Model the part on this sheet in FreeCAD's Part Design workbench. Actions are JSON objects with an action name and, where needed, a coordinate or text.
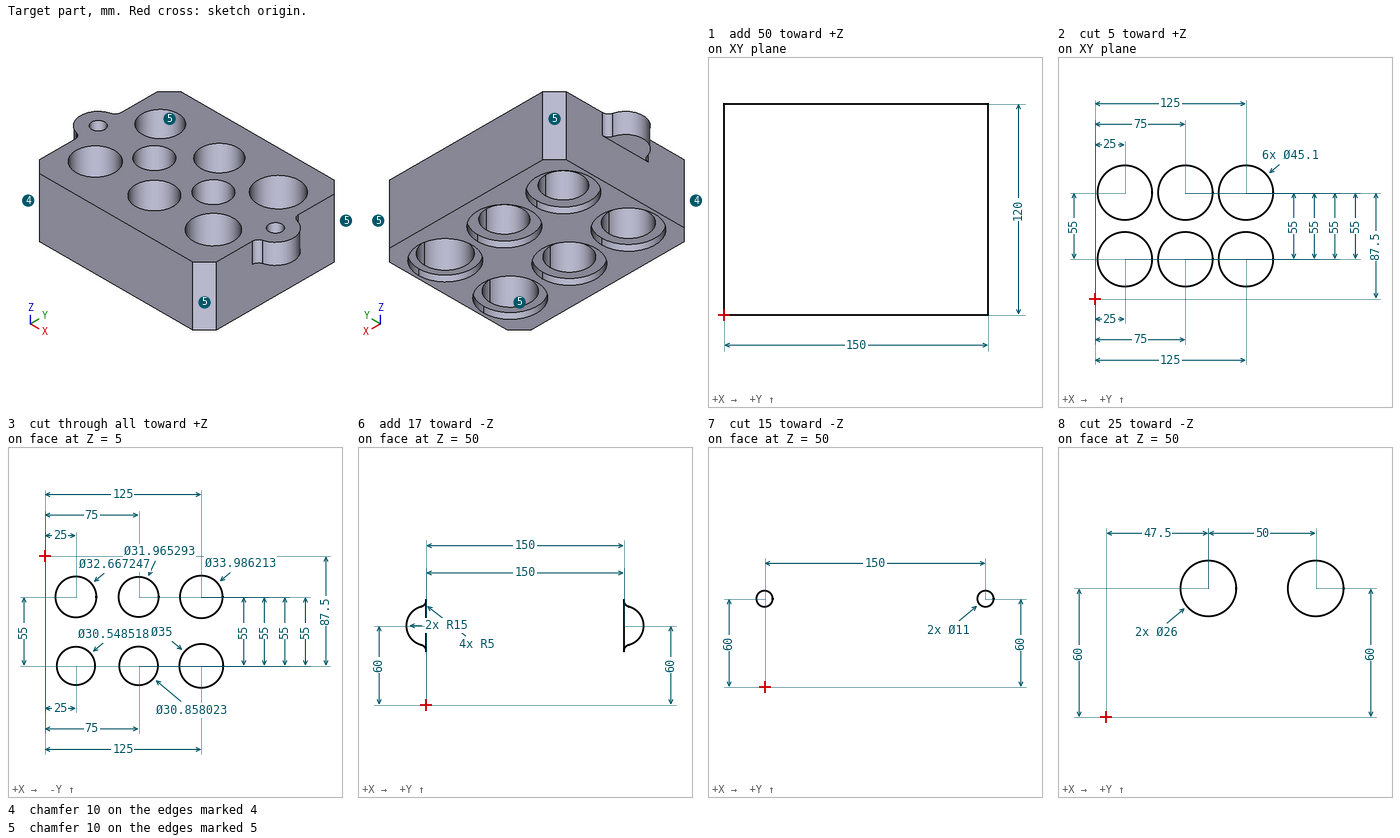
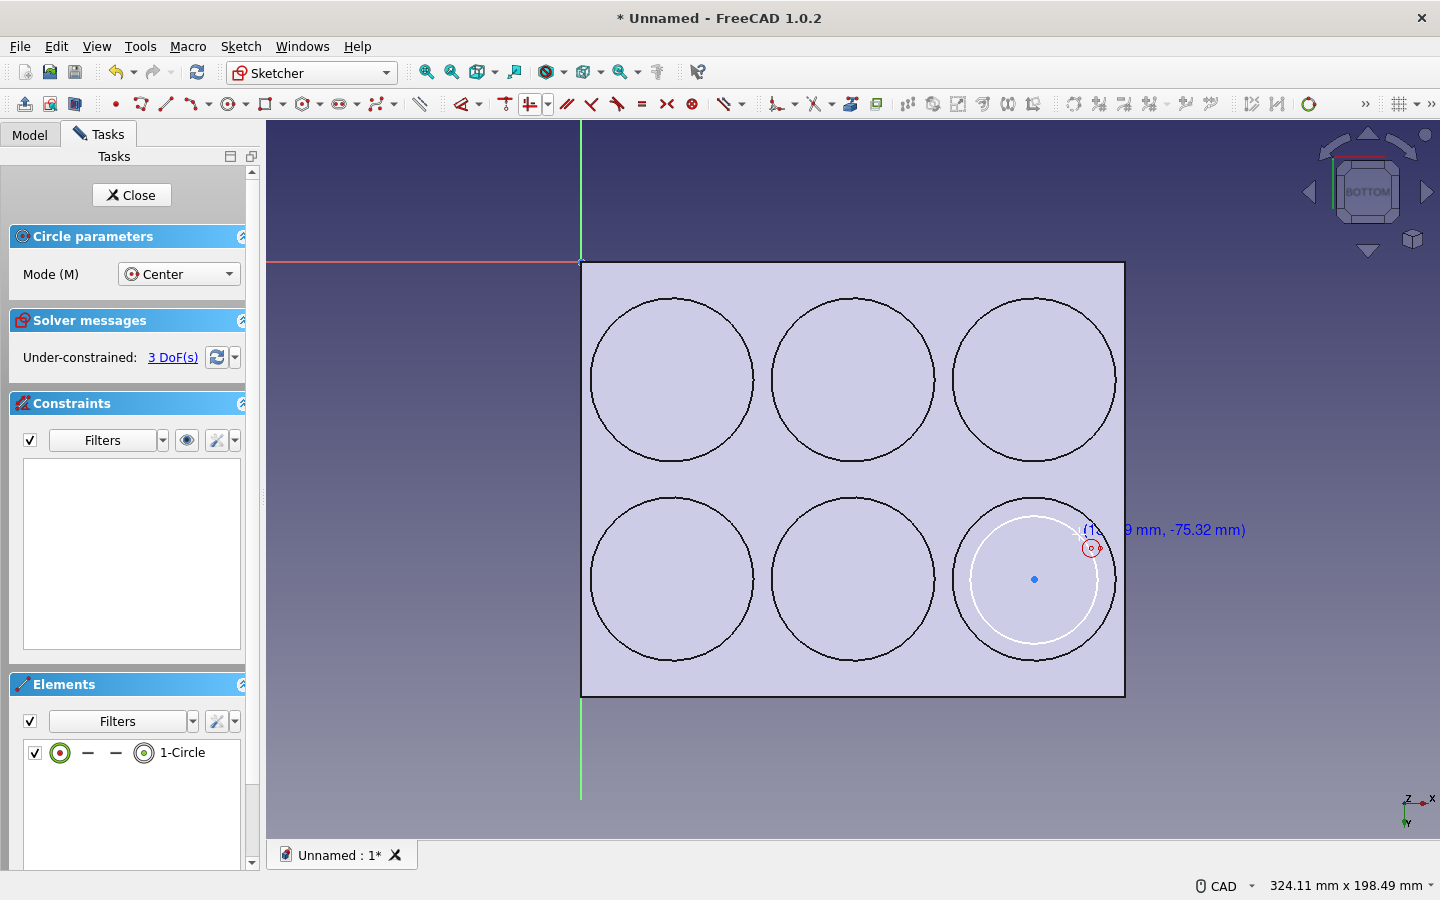
{"action": "left_click", "coordinate": [853, 579]}
{"action": "left_click", "coordinate": [893, 540]}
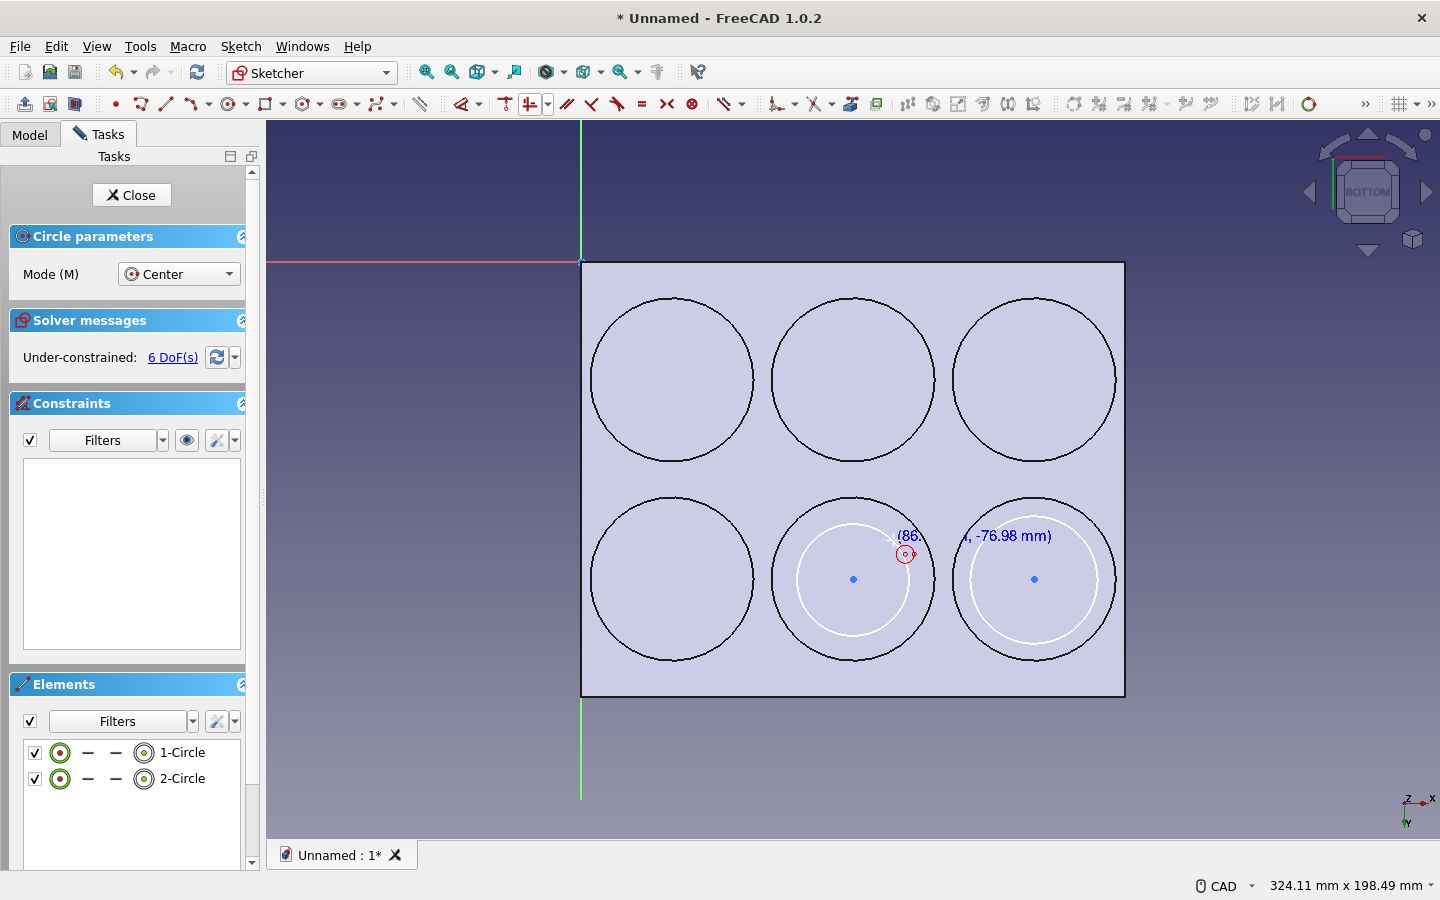
{"action": "left_click", "coordinate": [672, 579]}
{"action": "left_click", "coordinate": [711, 540]}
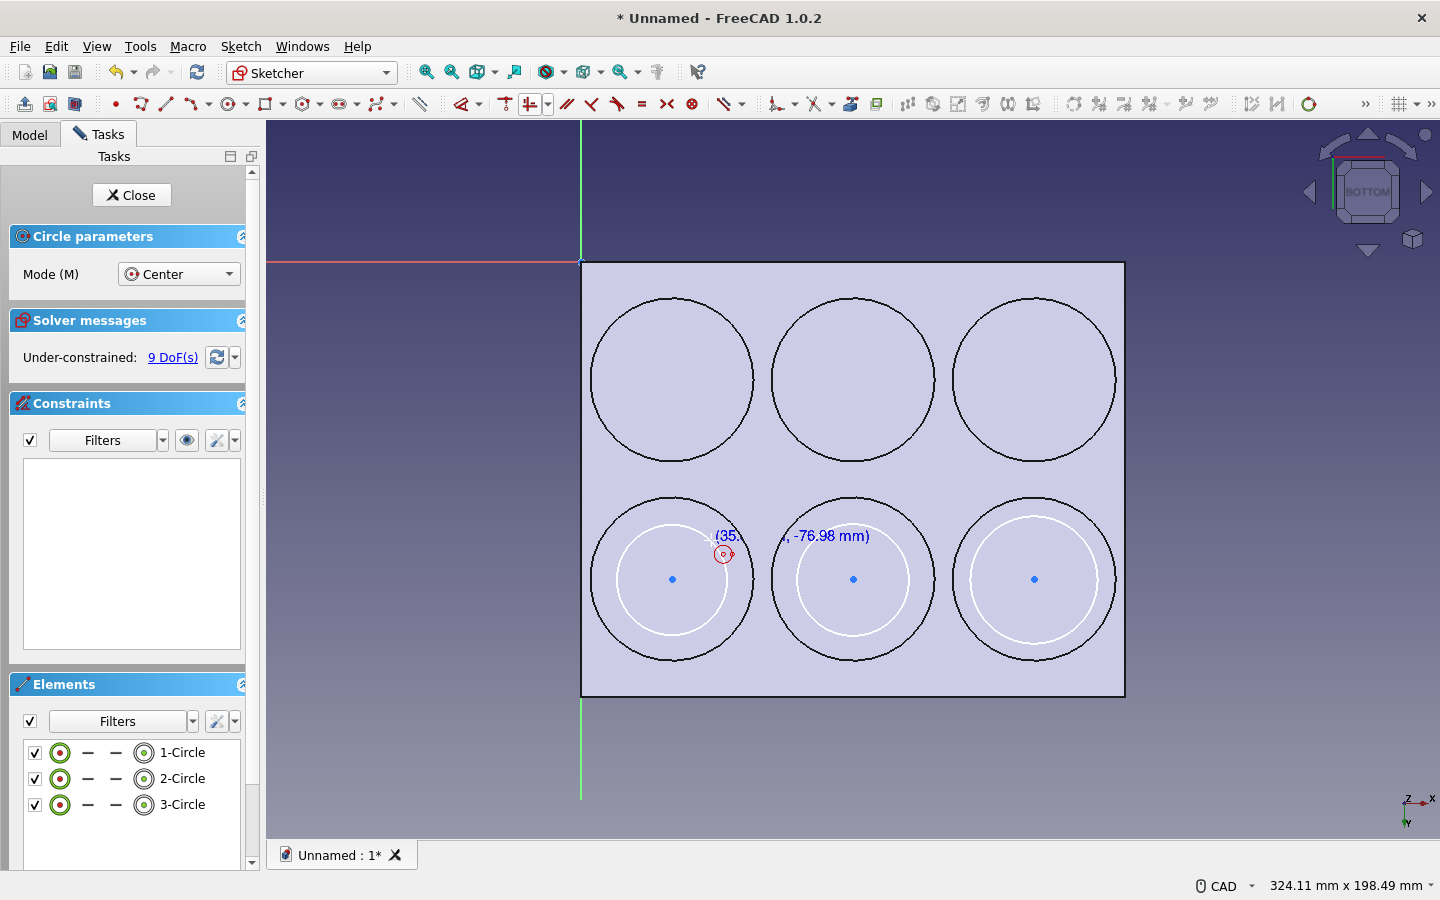
{"action": "left_click", "coordinate": [1034, 380]}
{"action": "left_click", "coordinate": [1078, 336]}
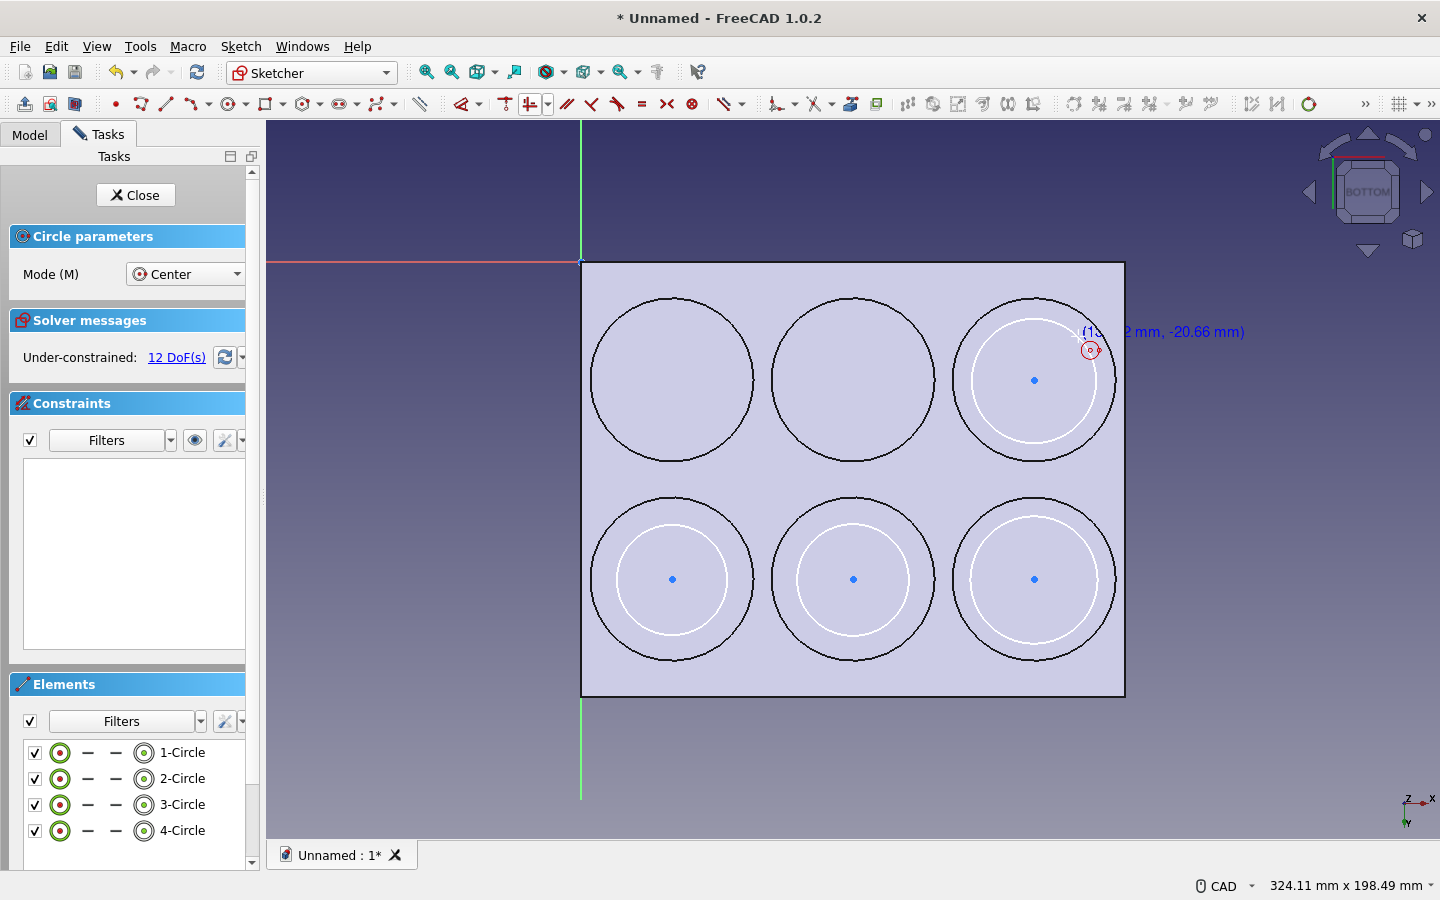
{"action": "left_click", "coordinate": [853, 380]}
{"action": "left_click", "coordinate": [894, 339]}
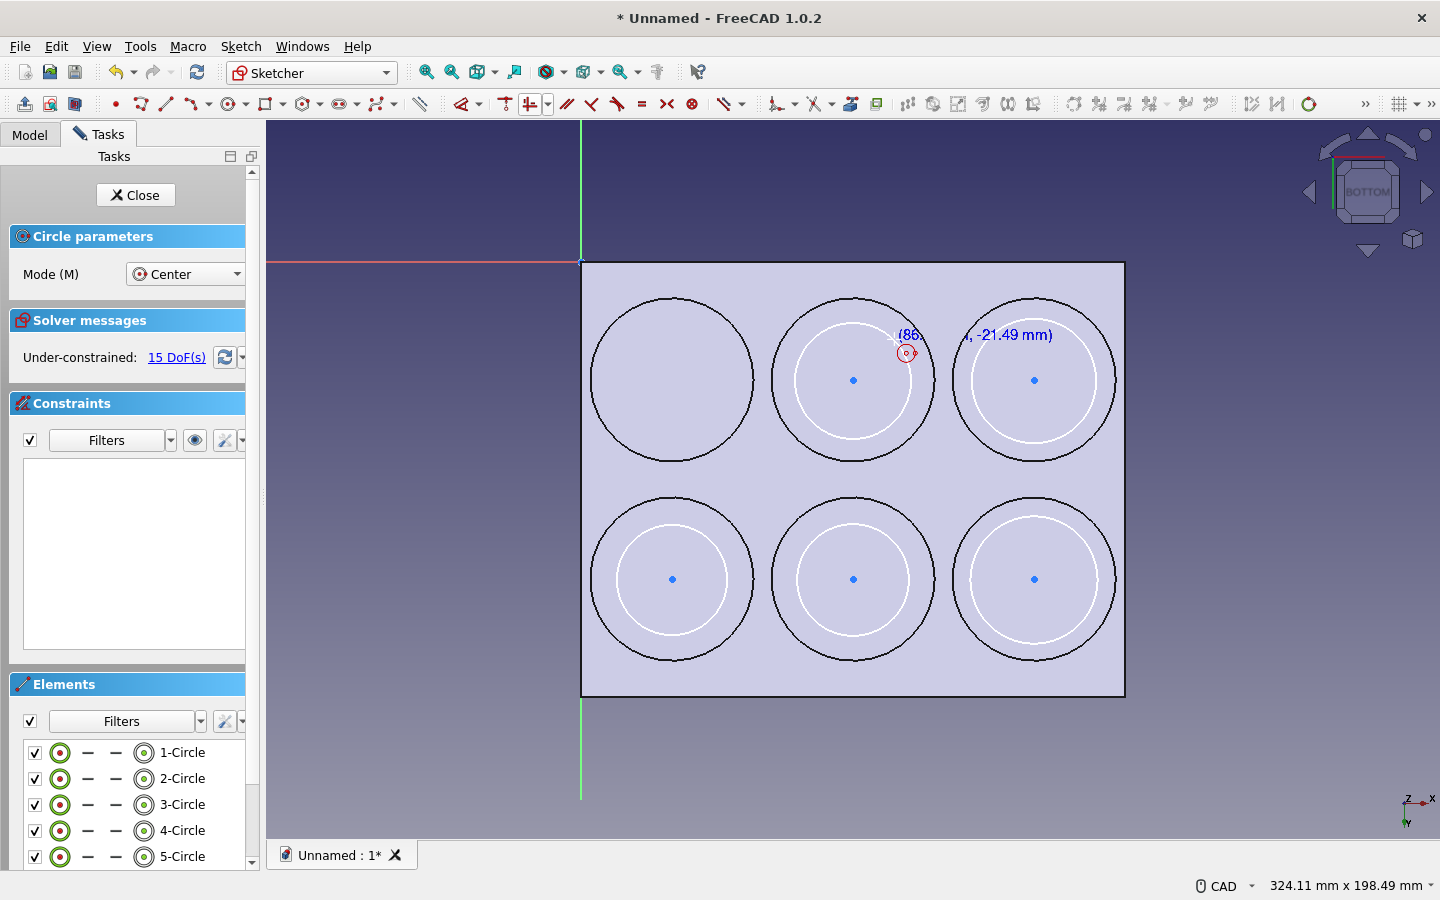
{"action": "left_click", "coordinate": [672, 380]}
{"action": "left_click", "coordinate": [714, 338]}
{"action": "key", "text": "Escape"}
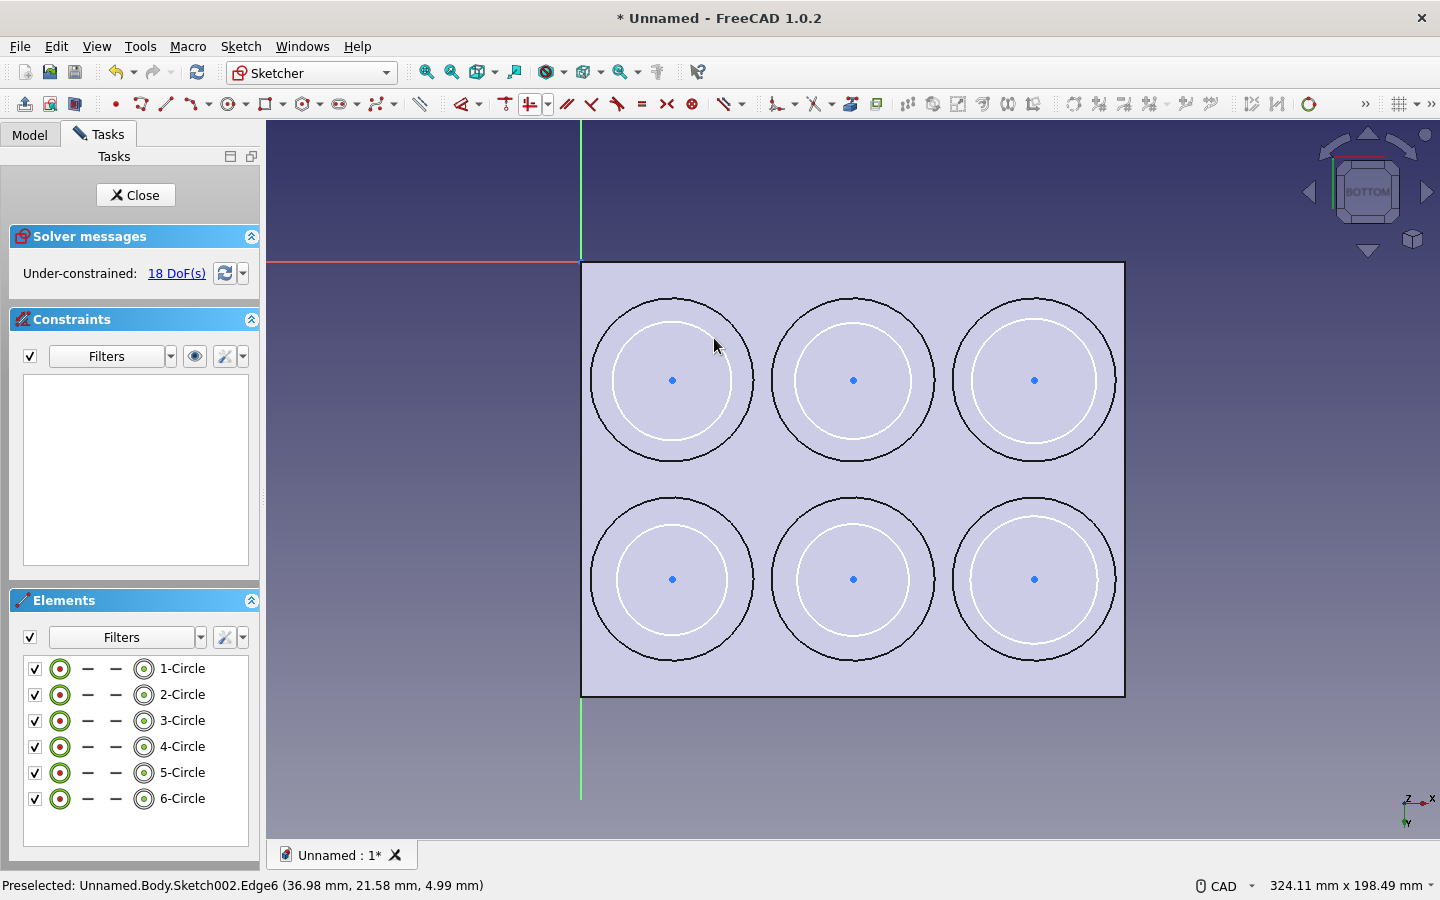
{"action": "key", "text": "d"}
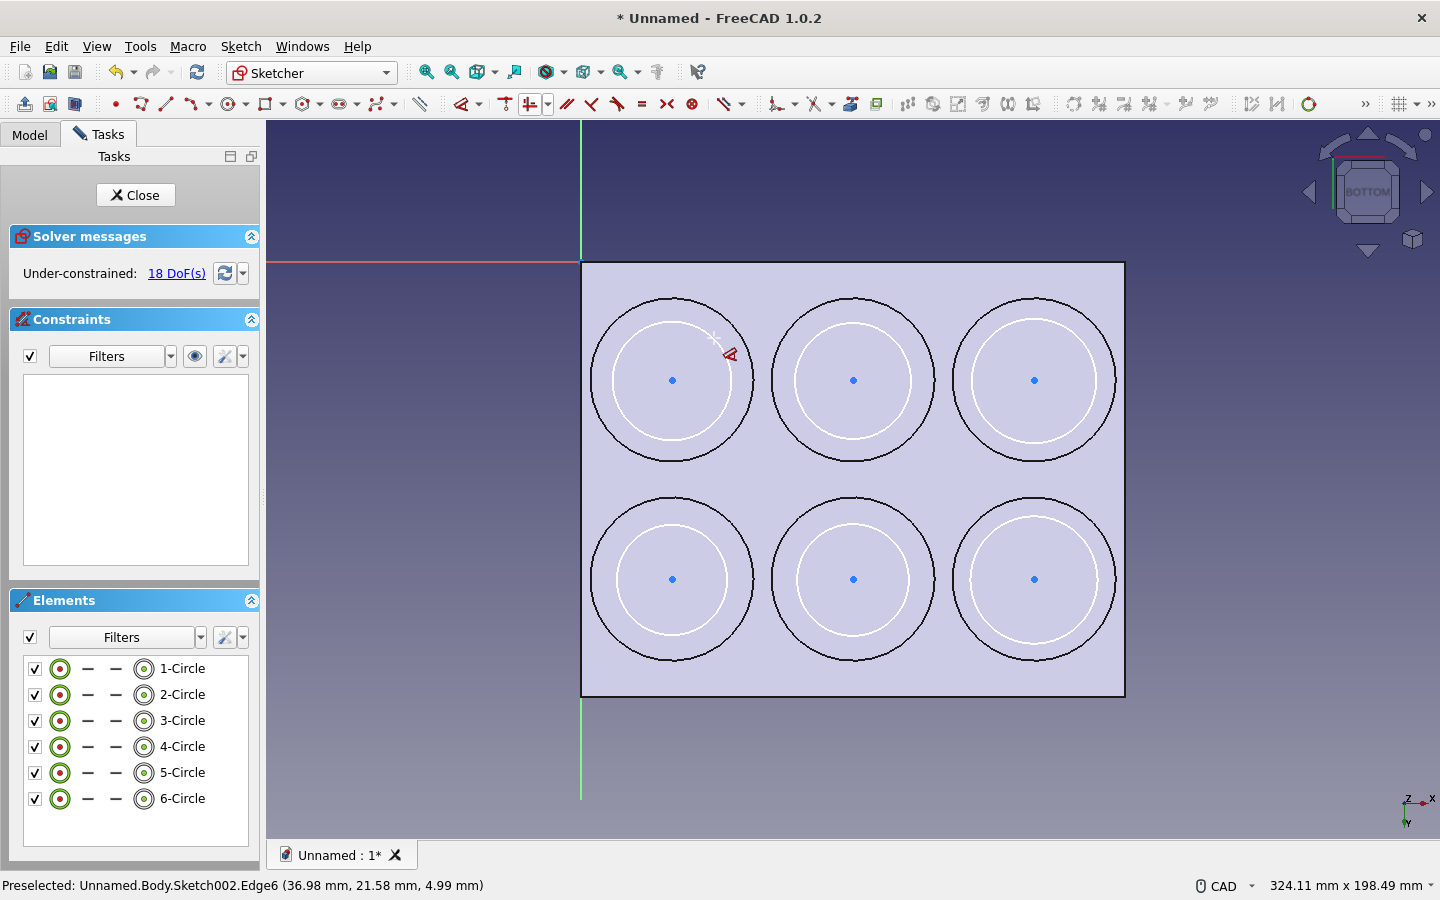
{"action": "left_click", "coordinate": [1079, 535]}
{"action": "left_click", "coordinate": [1102, 512]}